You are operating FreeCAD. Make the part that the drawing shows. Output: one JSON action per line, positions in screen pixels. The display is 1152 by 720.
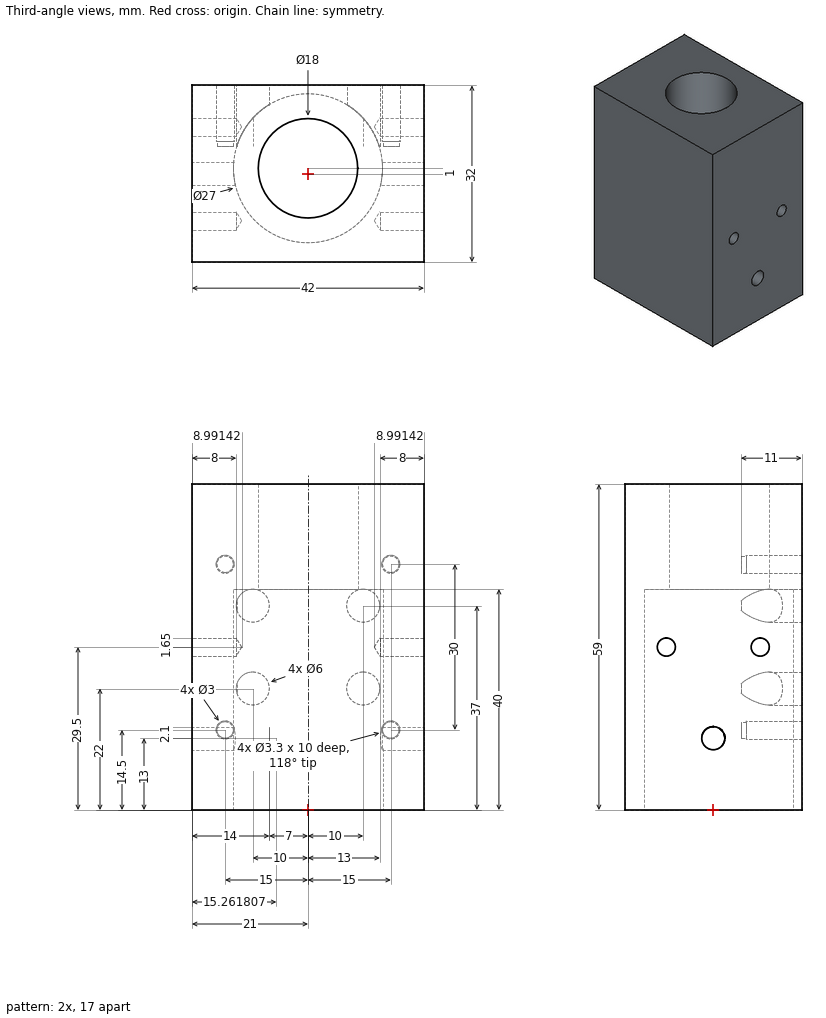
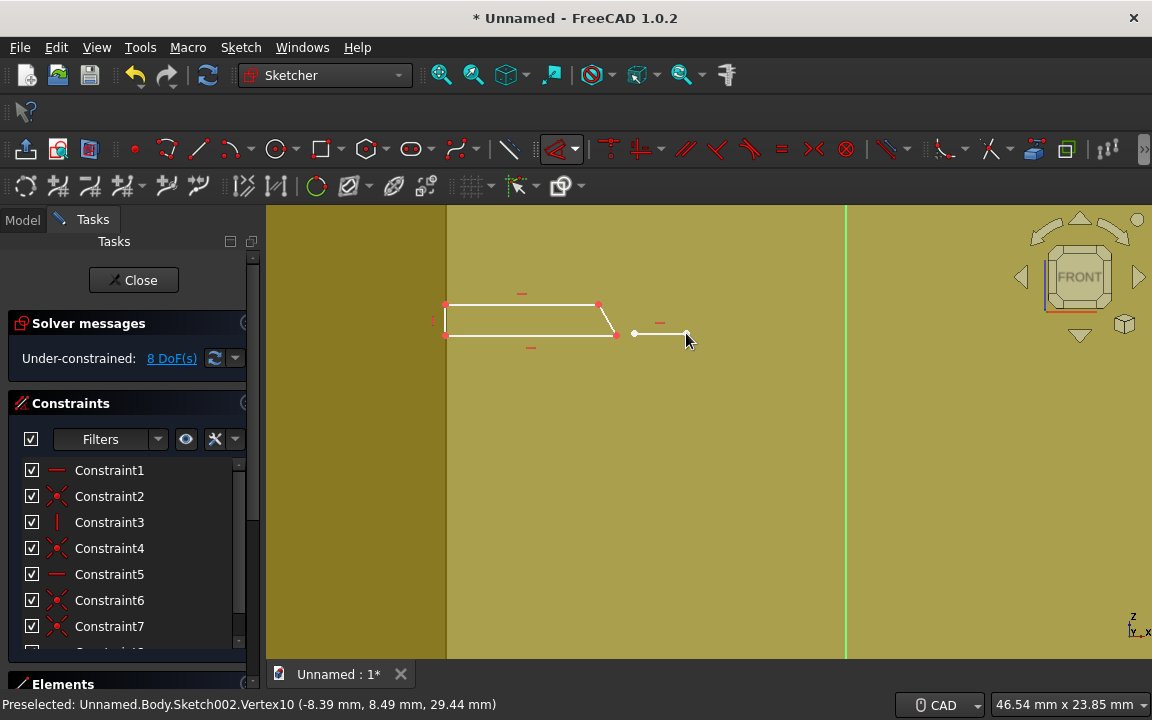
{"action": "left_click", "coordinate": [650, 334]}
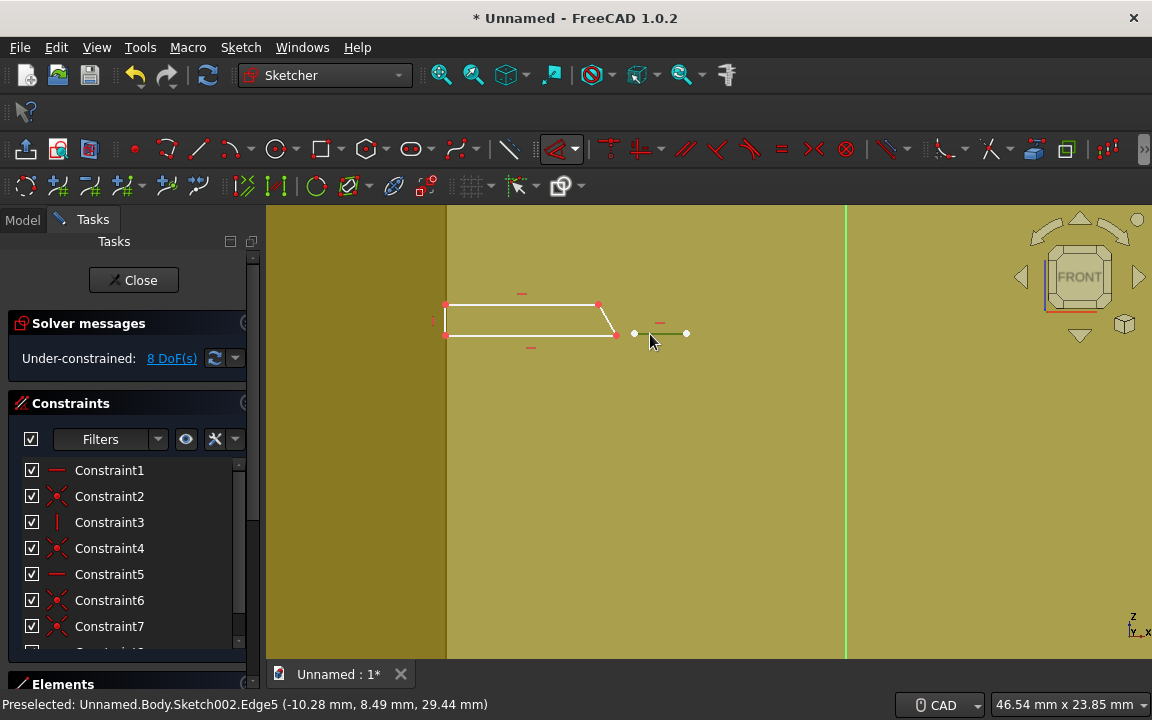
{"action": "key", "text": "g n"}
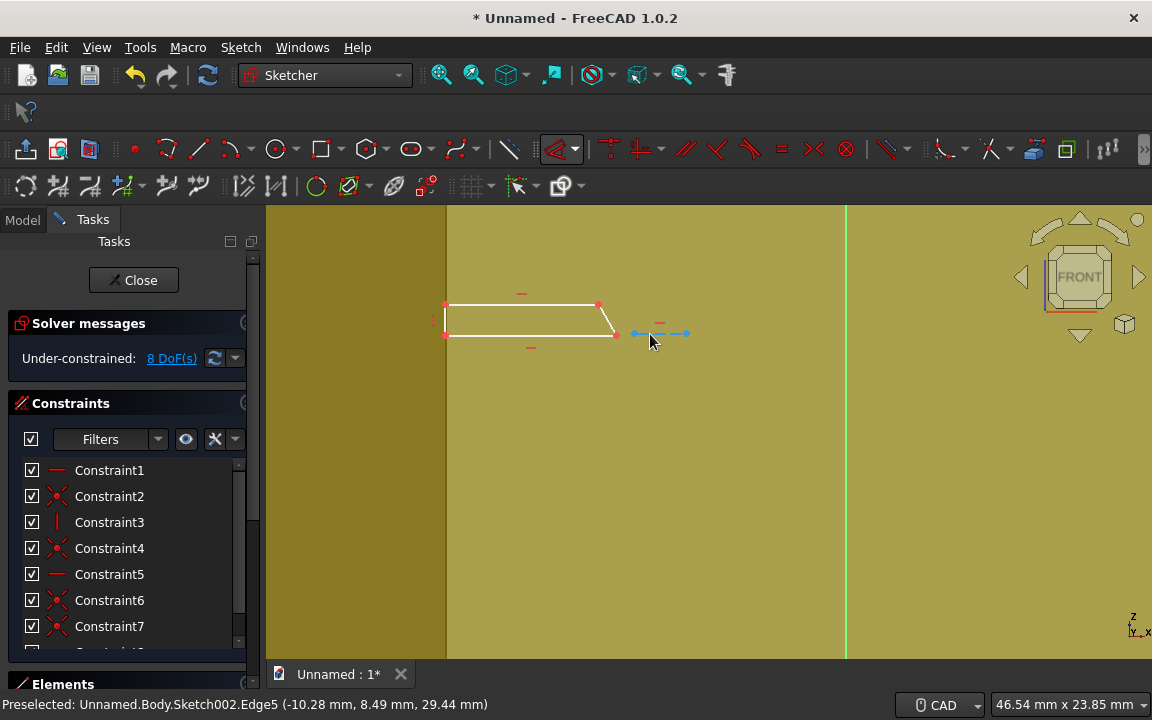
{"action": "left_click", "coordinate": [491, 305]}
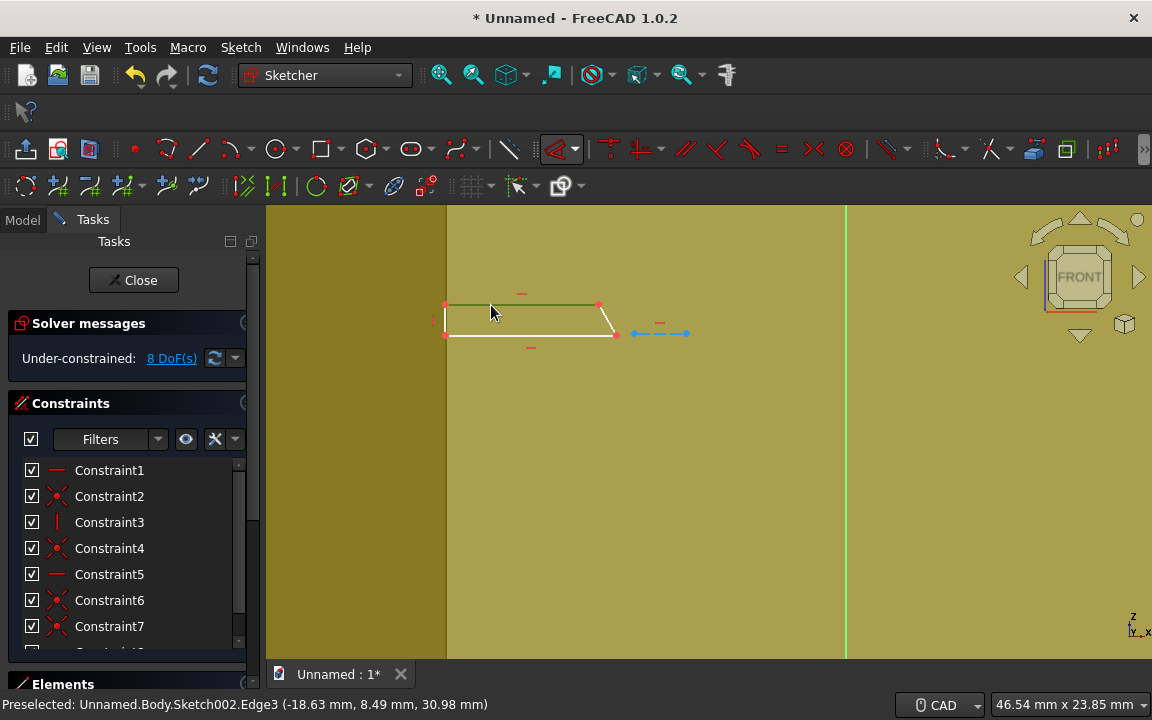
{"action": "key", "text": "l"}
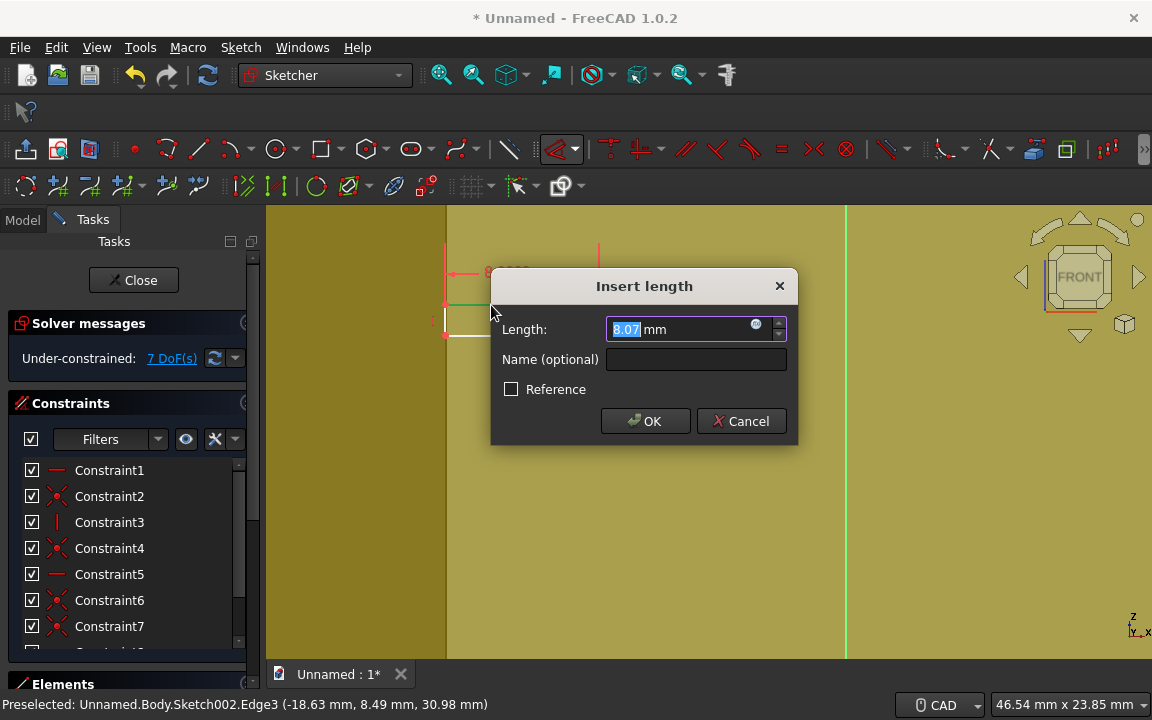
{"action": "type", "text": "8"}
{"action": "key", "text": "Return"}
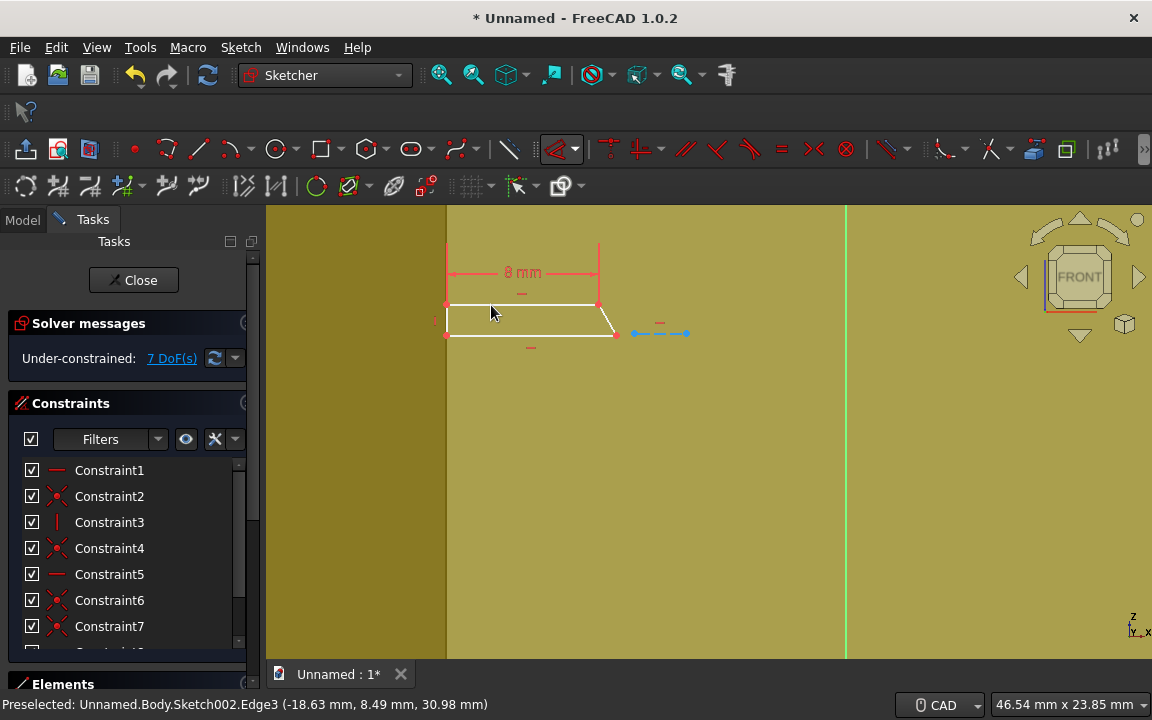
{"action": "left_click", "coordinate": [447, 336]}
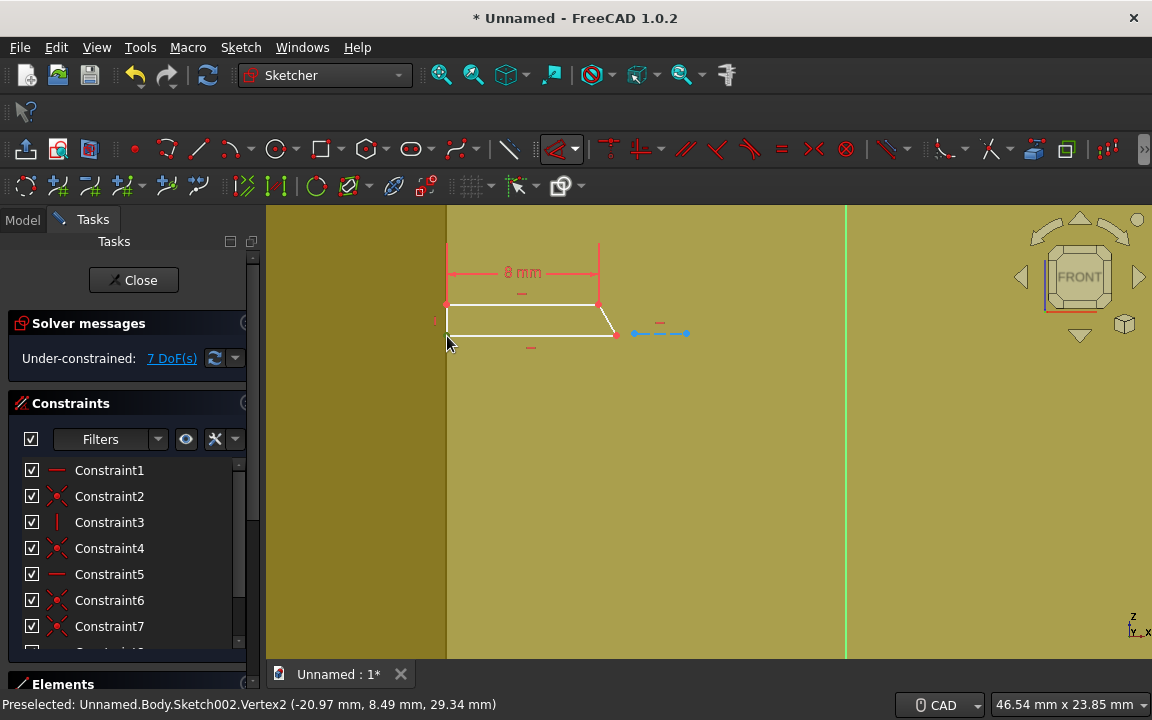
{"action": "left_click", "coordinate": [578, 150]}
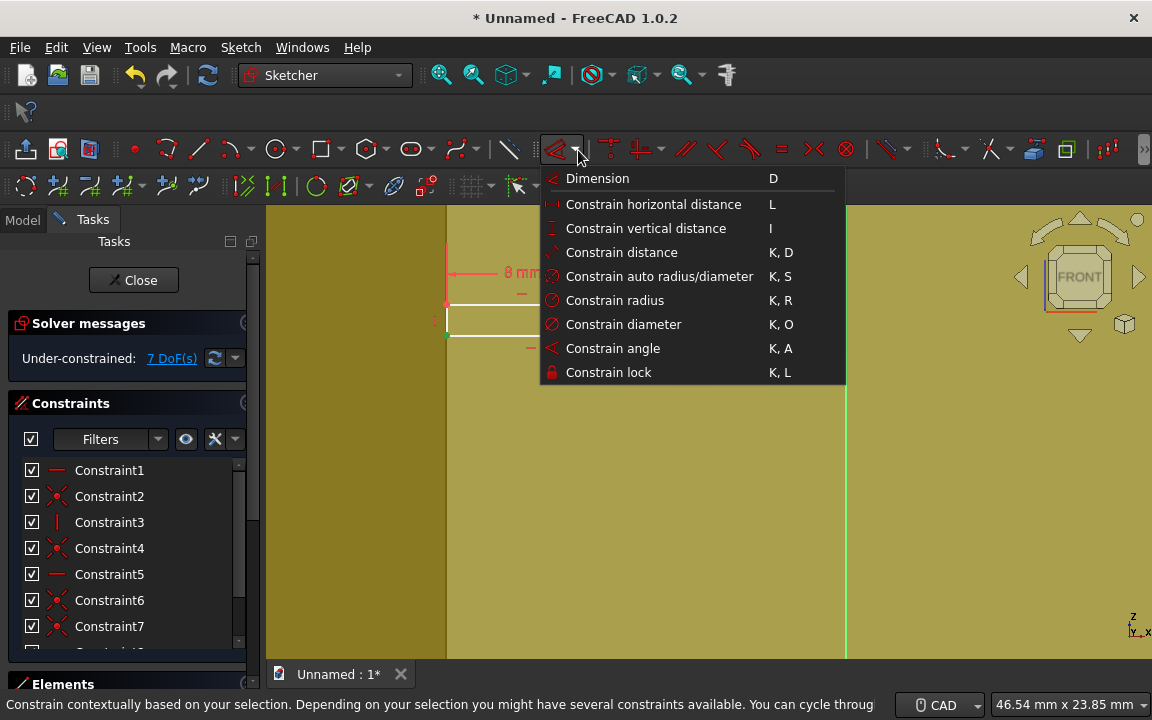
{"action": "left_click", "coordinate": [693, 204]}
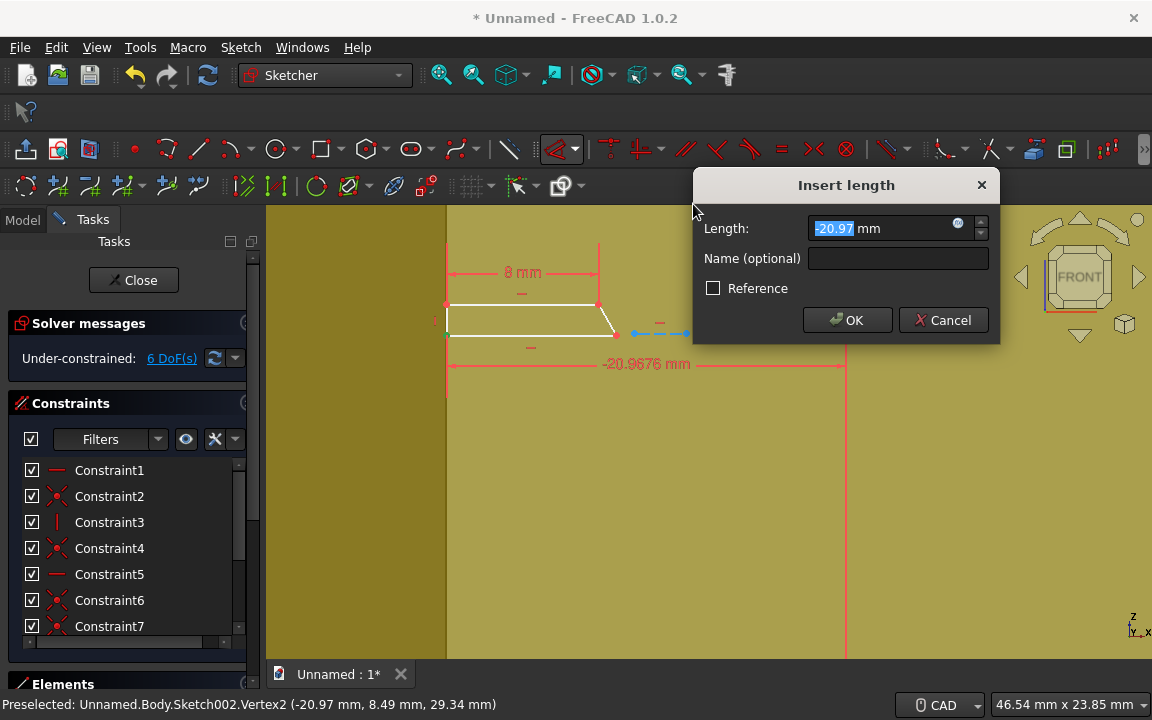
{"action": "type", "text": "-21"}
{"action": "key", "text": "Return"}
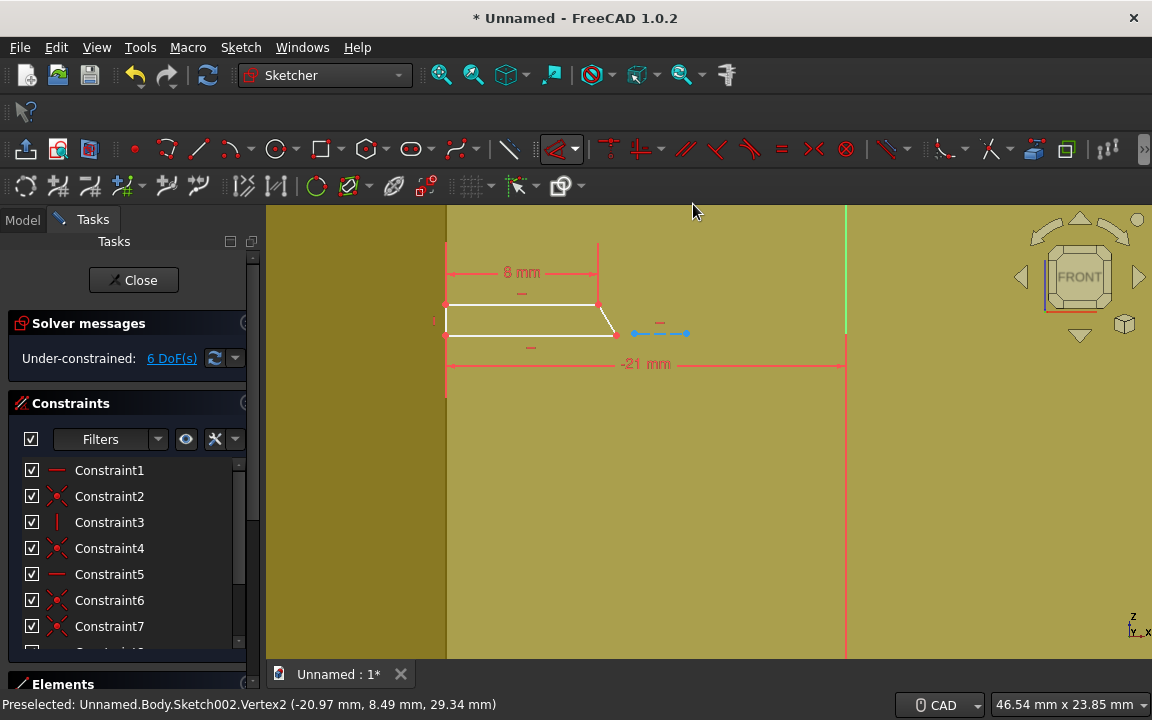
{"action": "scroll", "coordinate": [446, 327], "scroll_direction": "up", "scroll_amount": 2}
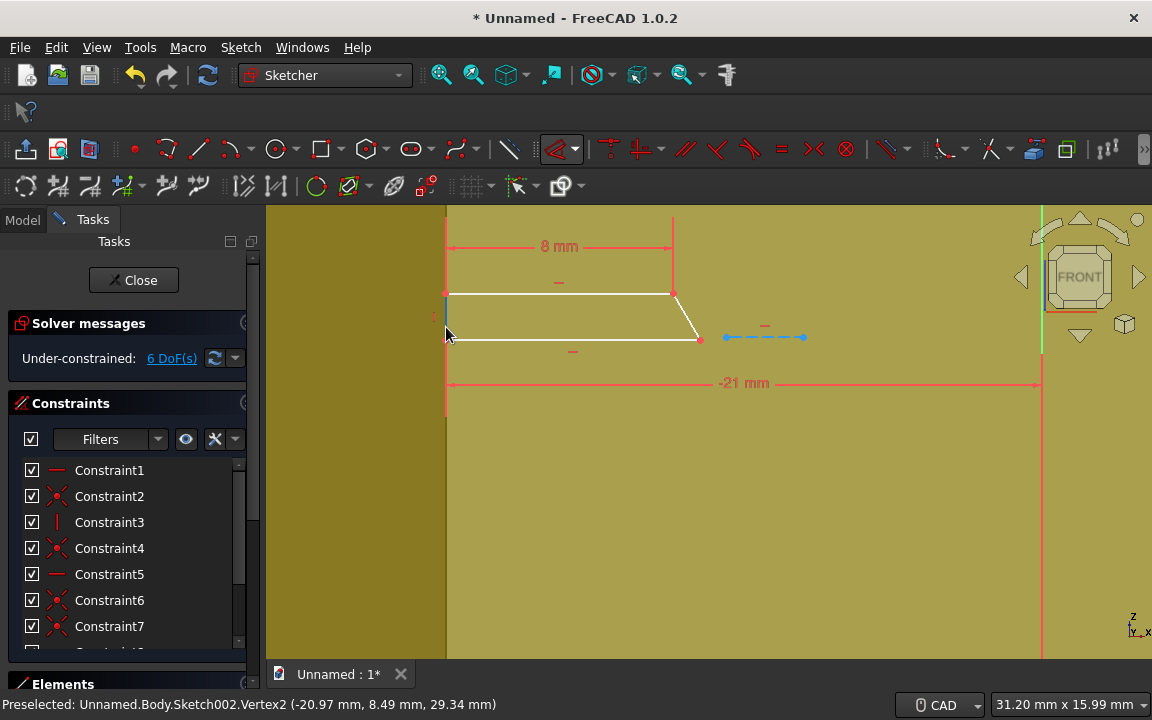
{"action": "left_click", "coordinate": [446, 326]}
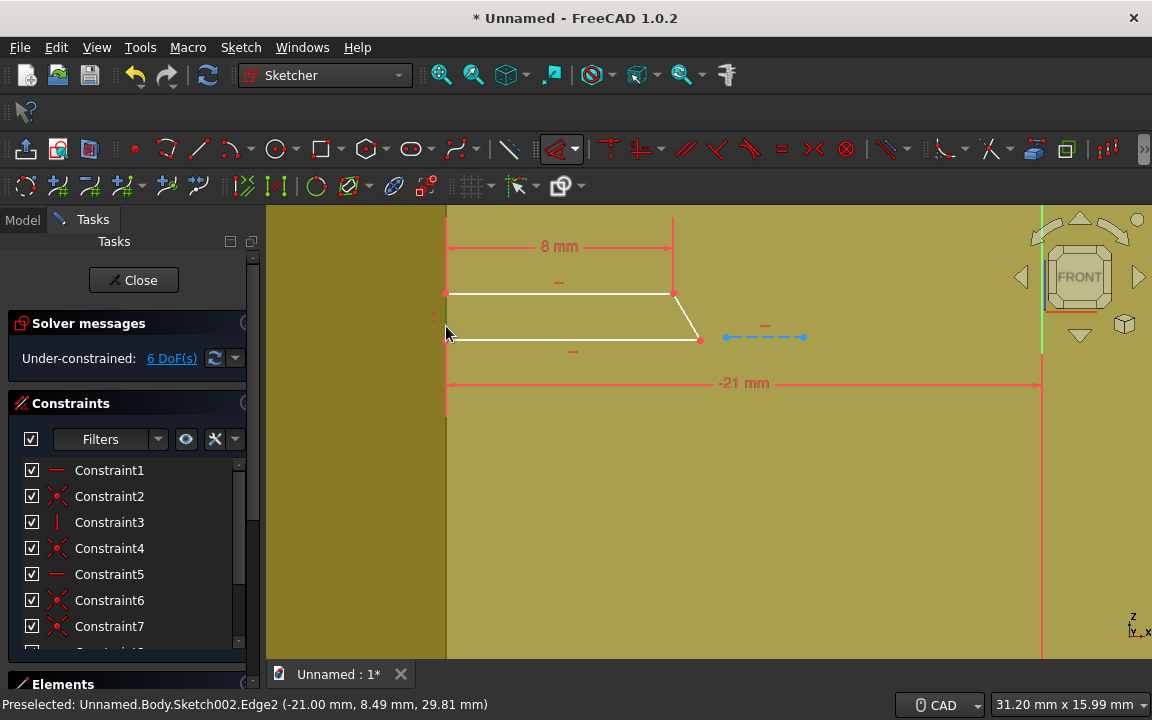
{"action": "left_click", "coordinate": [578, 150]}